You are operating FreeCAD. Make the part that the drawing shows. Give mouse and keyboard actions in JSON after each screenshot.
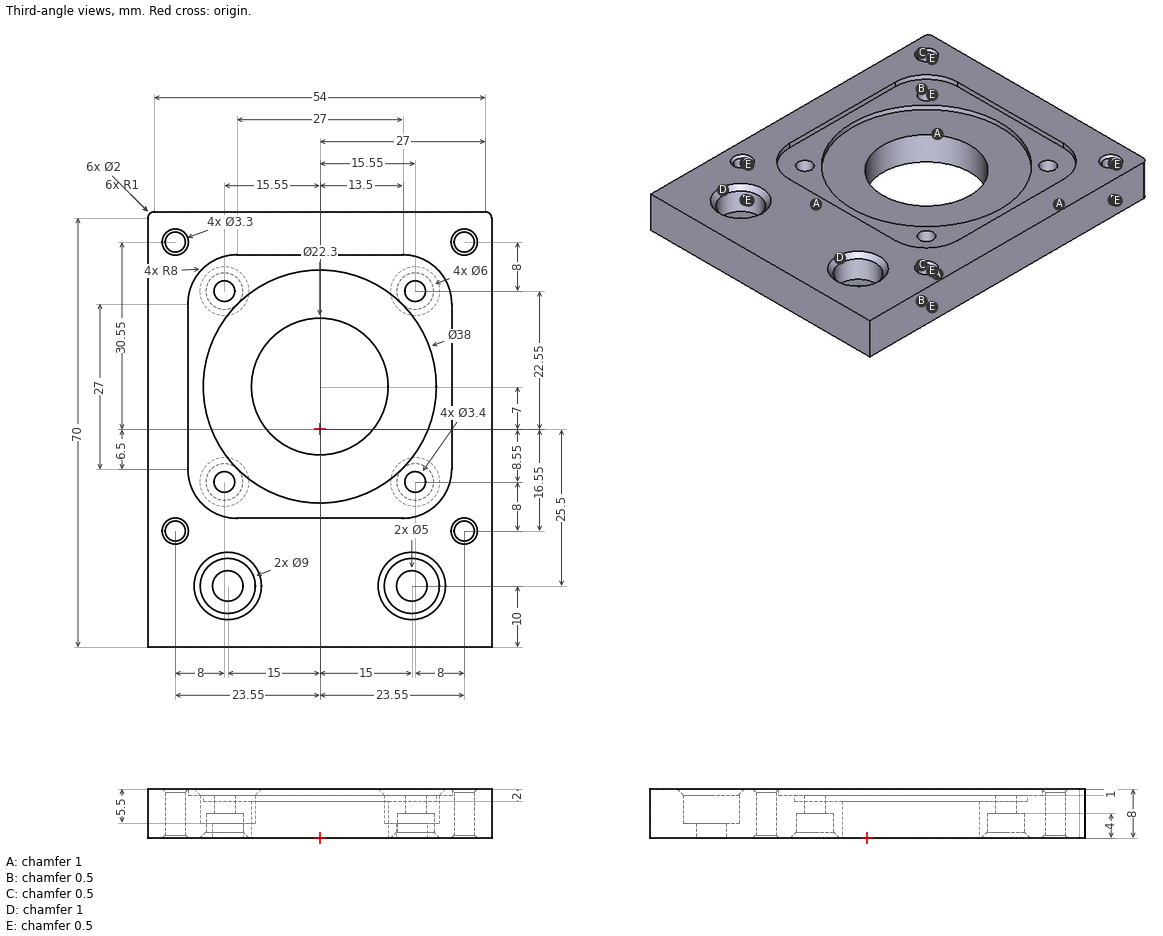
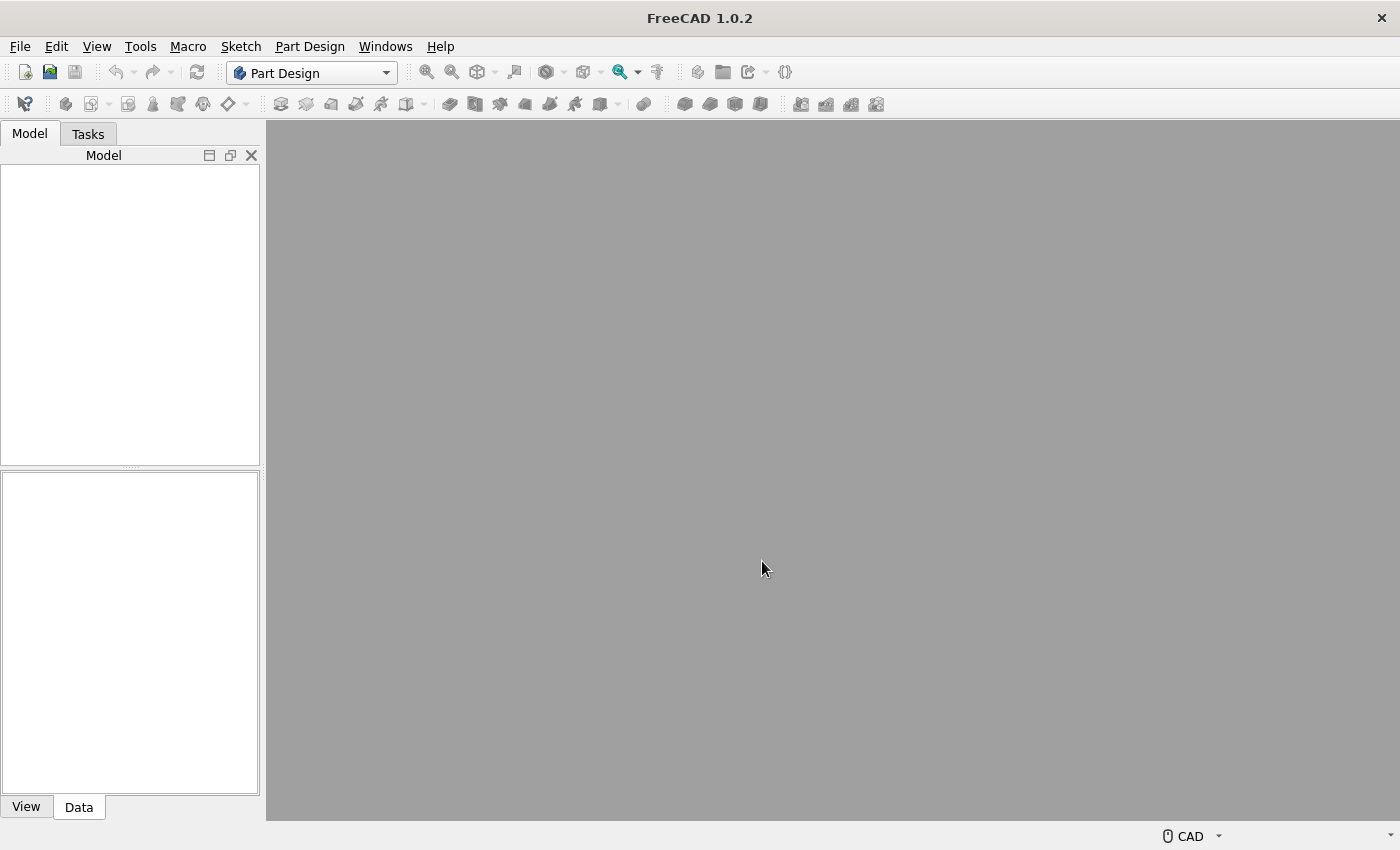
{"action": "left_click", "coordinate": [25, 72]}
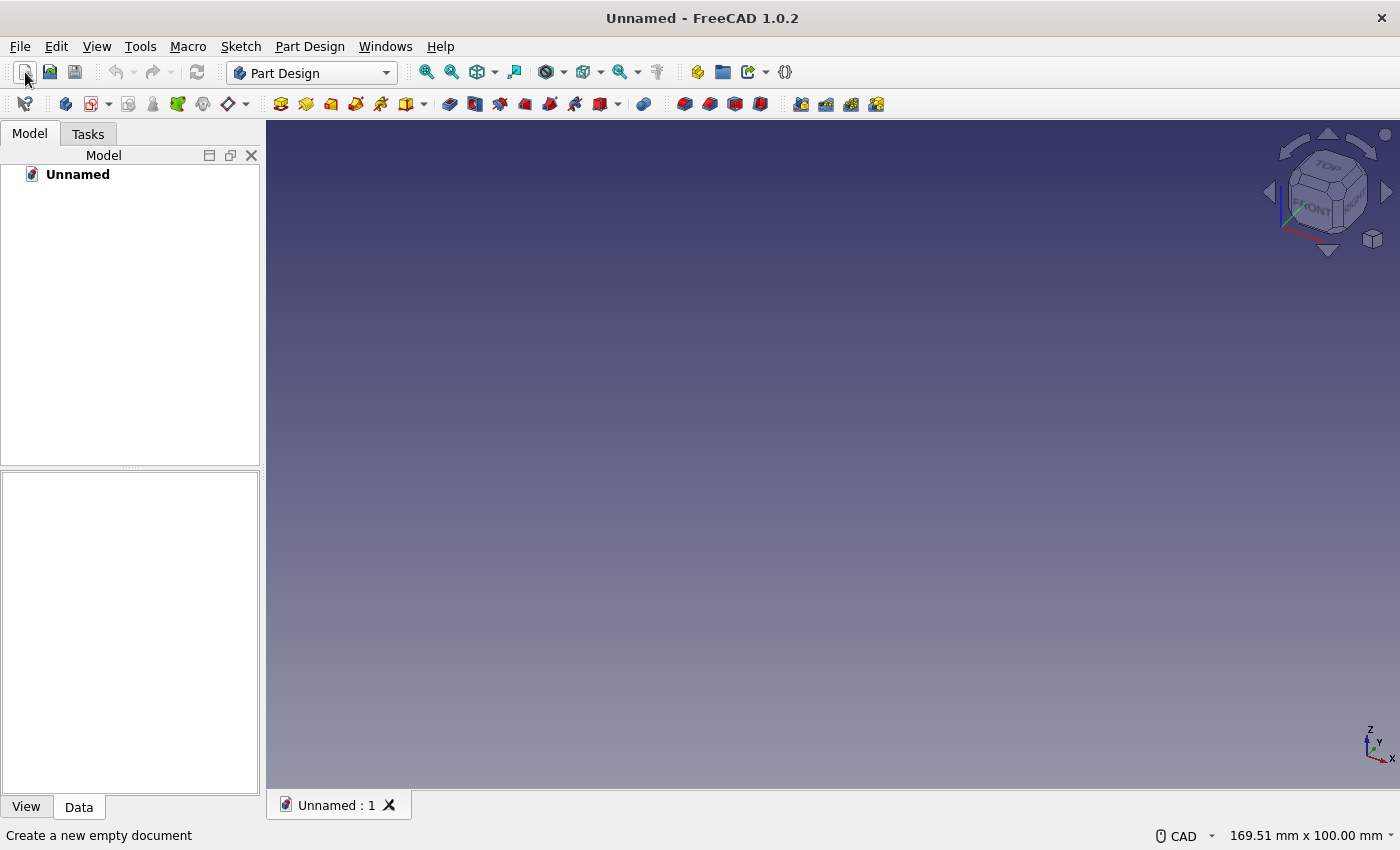
{"action": "left_click", "coordinate": [90, 104]}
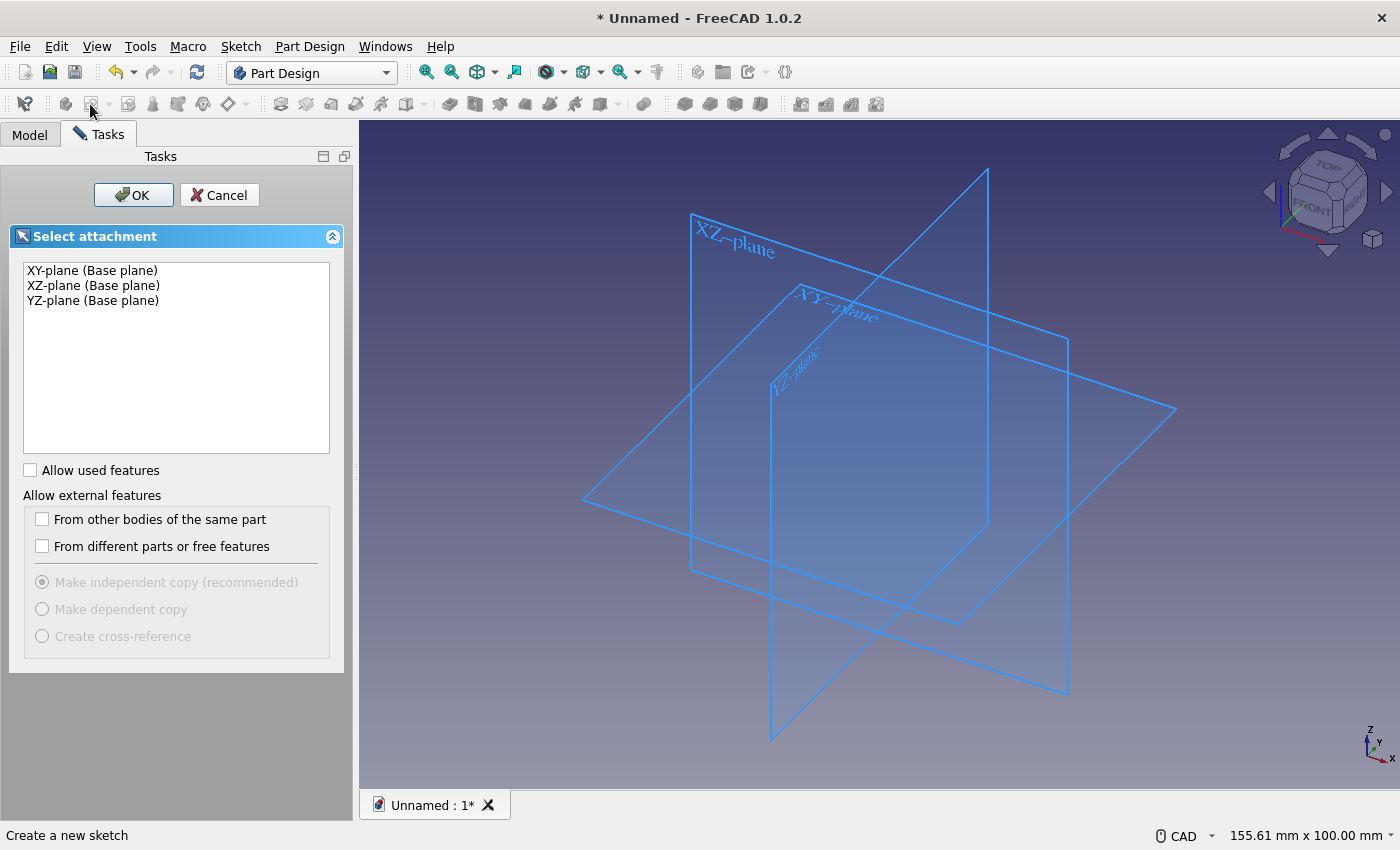
{"action": "left_click", "coordinate": [84, 270]}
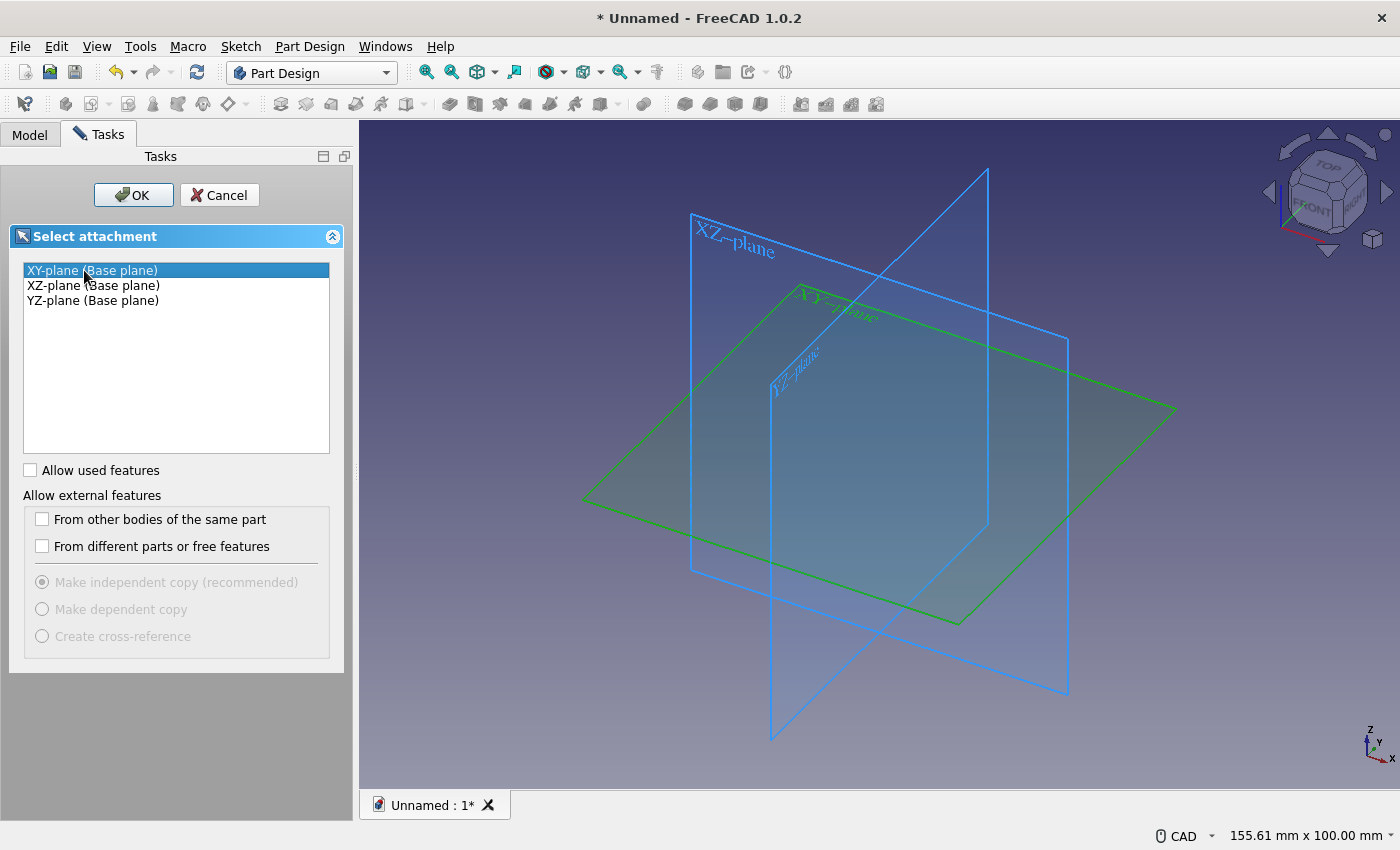
{"action": "left_click", "coordinate": [134, 195]}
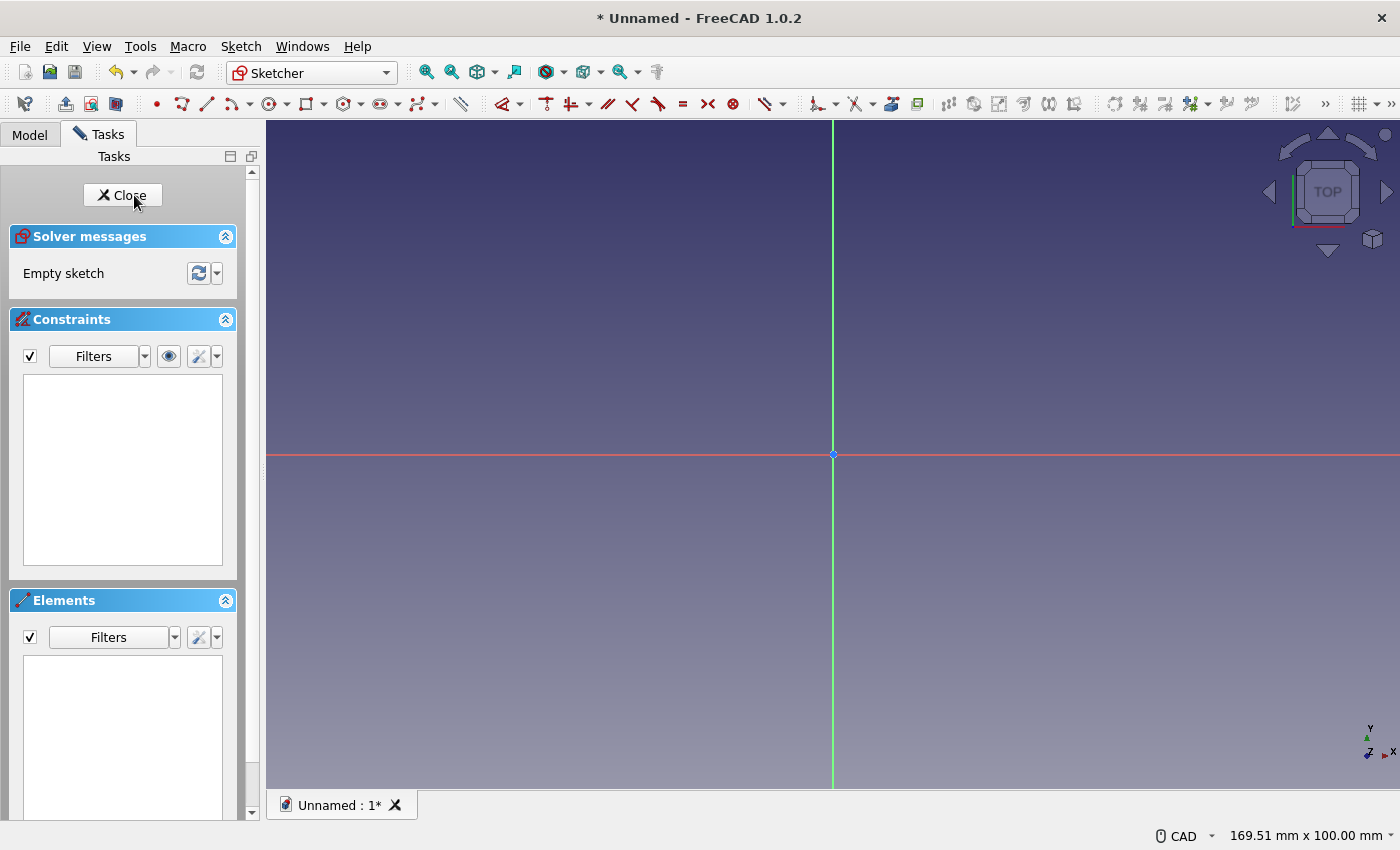
{"action": "key", "text": "g l"}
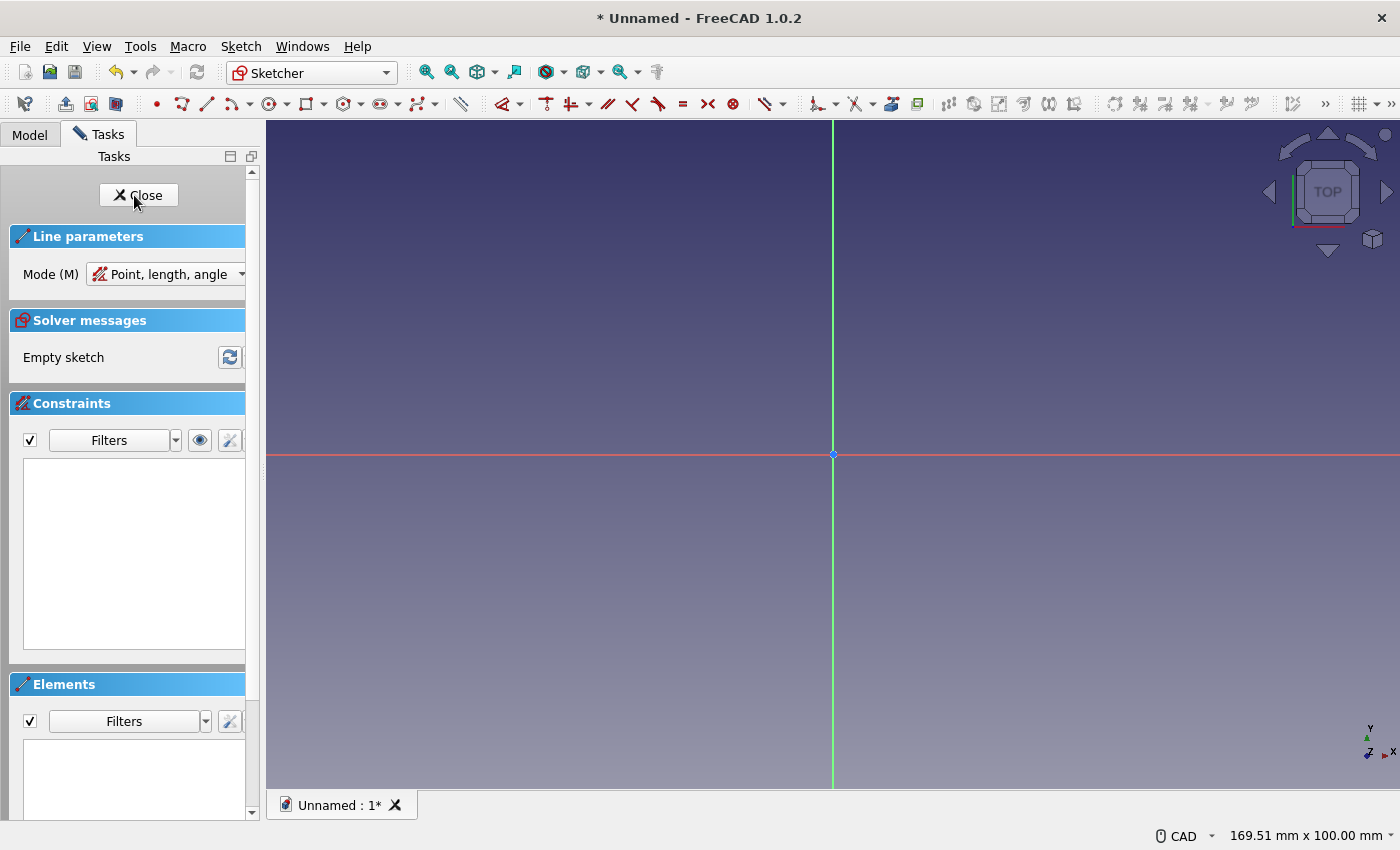
{"action": "left_click", "coordinate": [1014, 217]}
{"action": "left_click", "coordinate": [652, 217]}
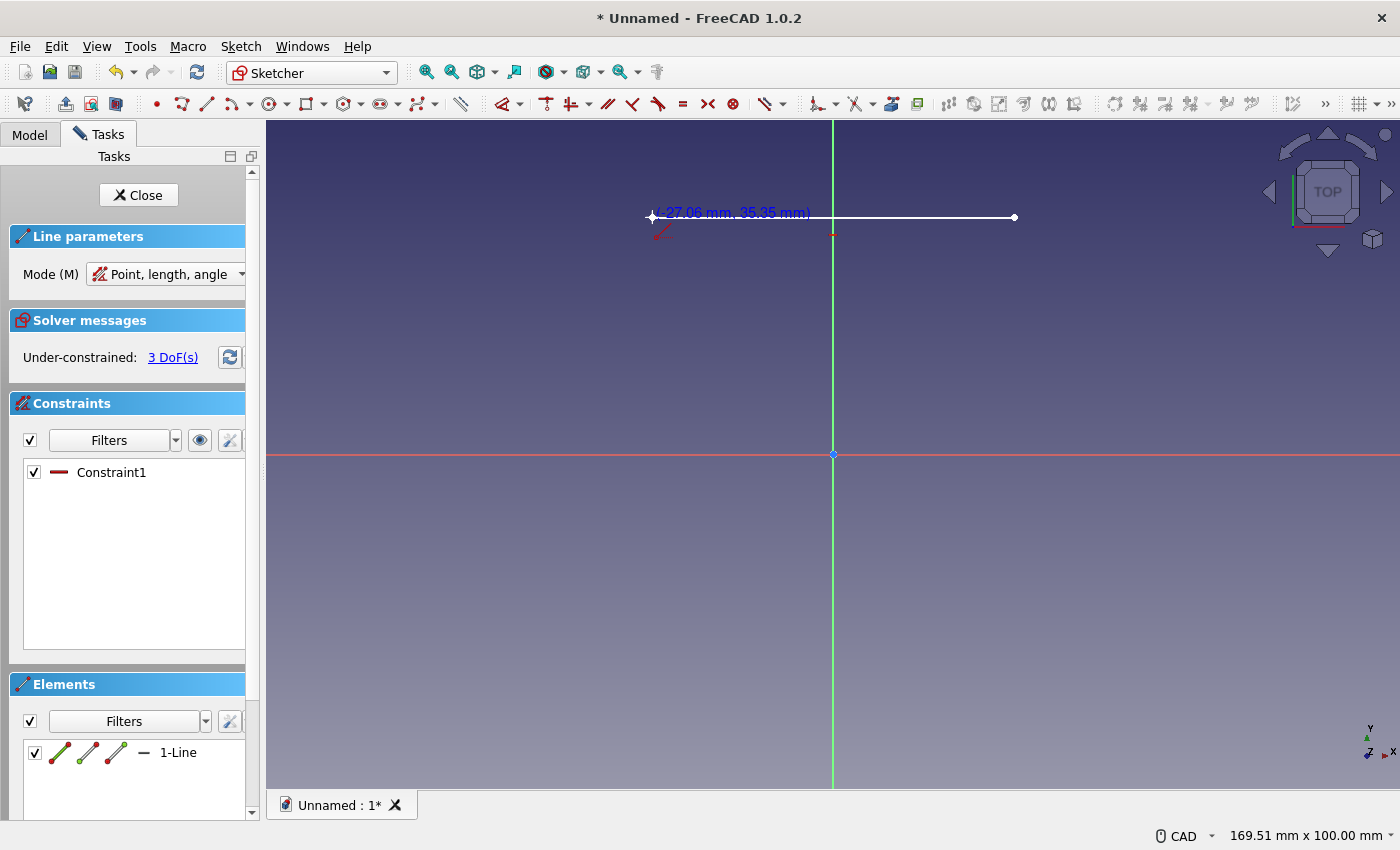
{"action": "key", "text": "g m"}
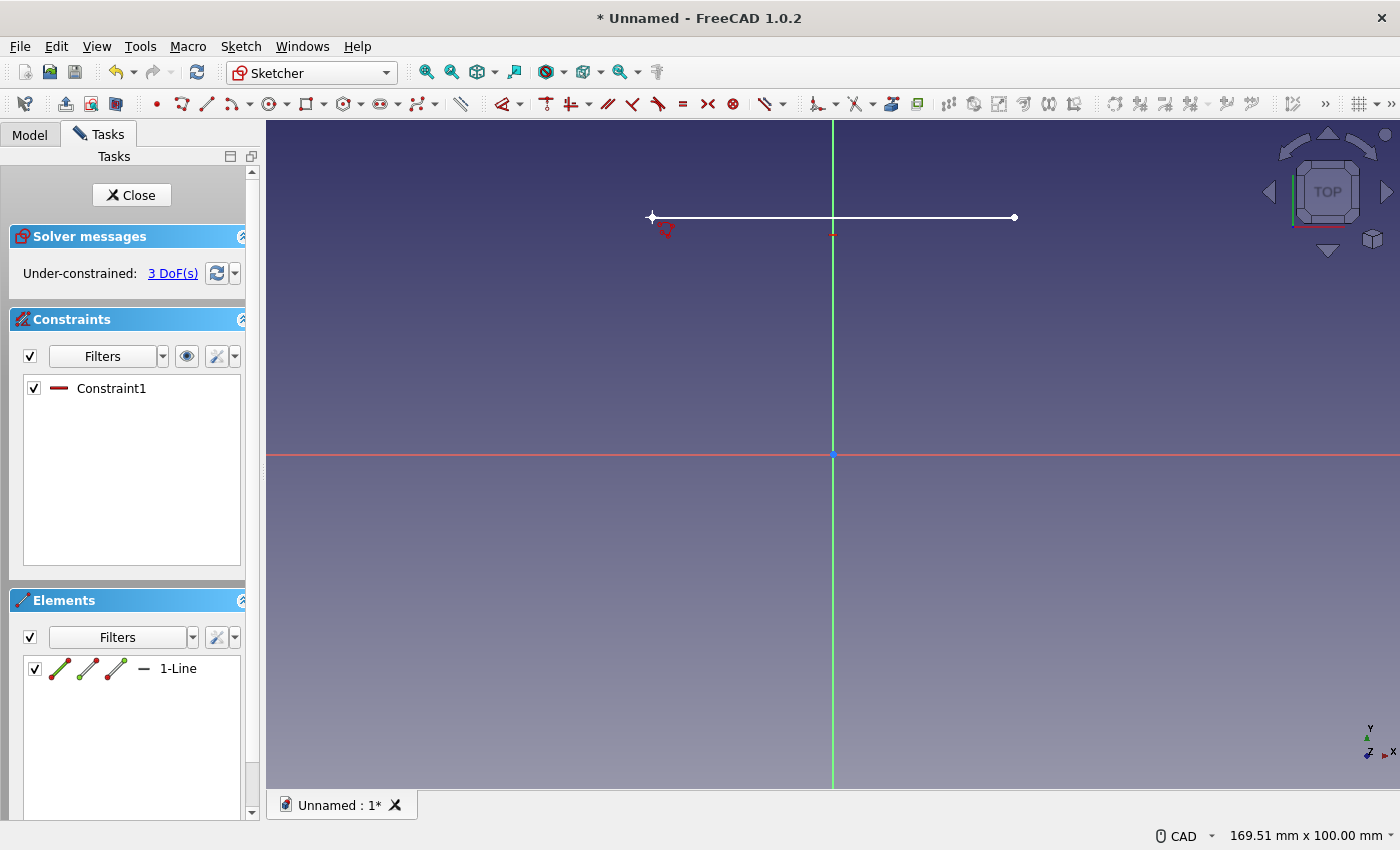
{"action": "scroll", "coordinate": [646, 224], "scroll_direction": "up", "scroll_amount": 3}